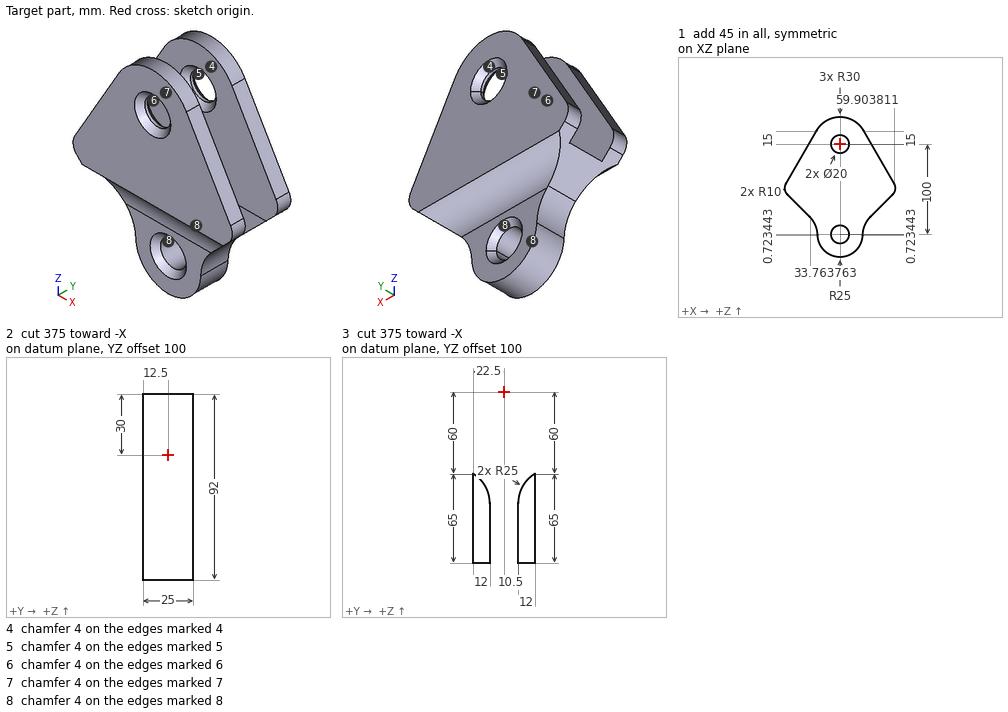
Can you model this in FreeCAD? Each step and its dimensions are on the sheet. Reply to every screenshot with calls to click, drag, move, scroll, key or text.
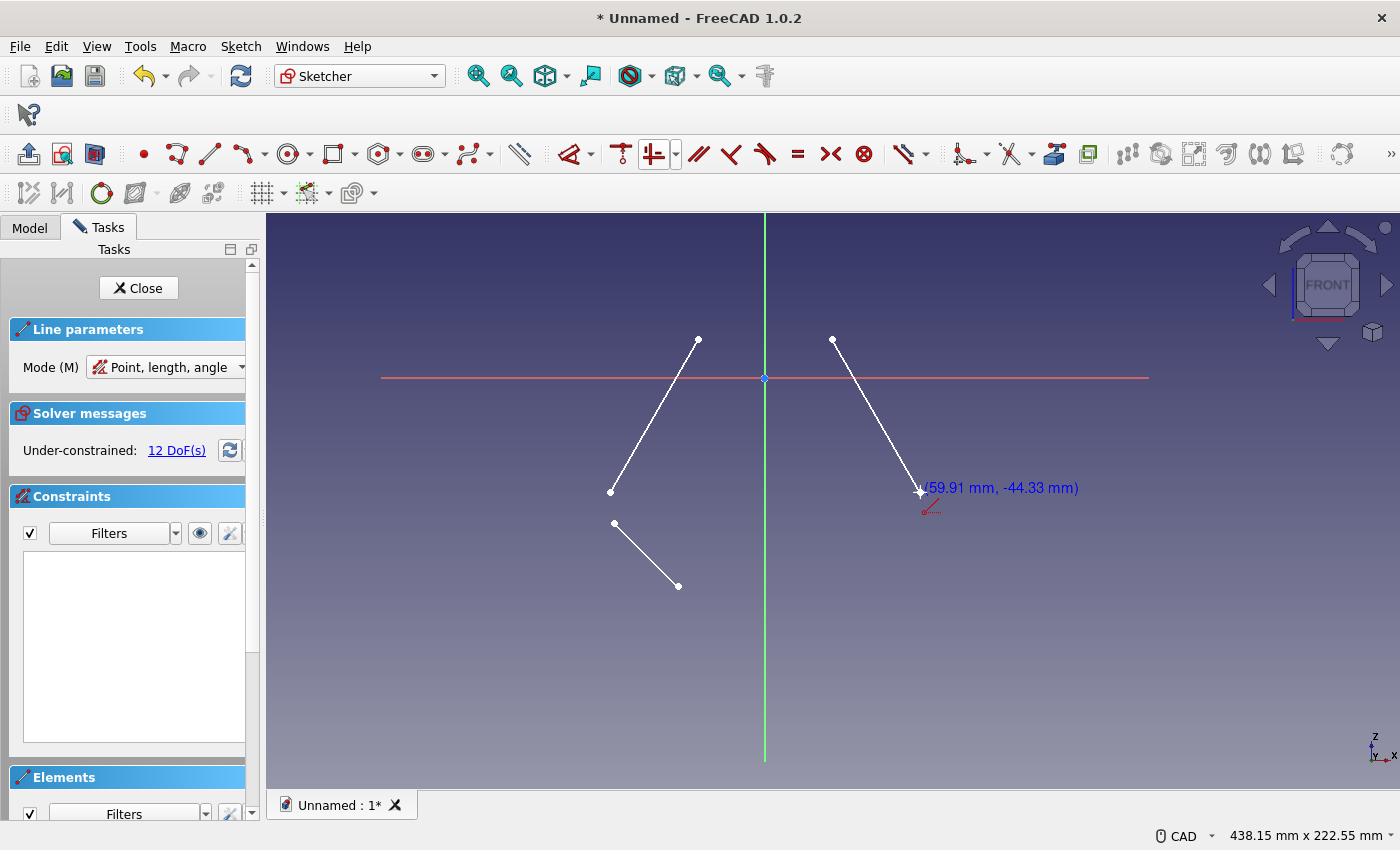
click(916, 523)
click(852, 586)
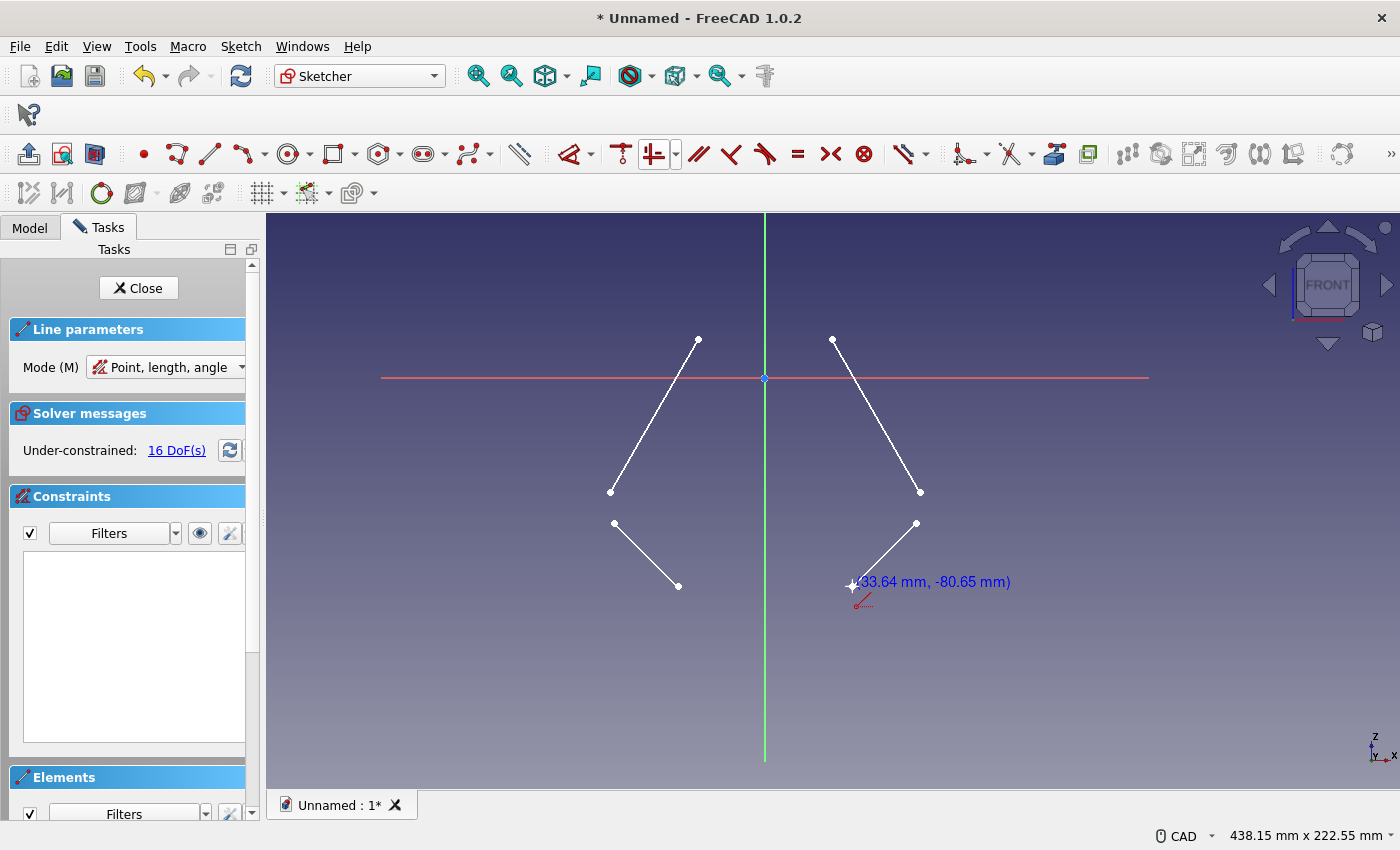
click(242, 154)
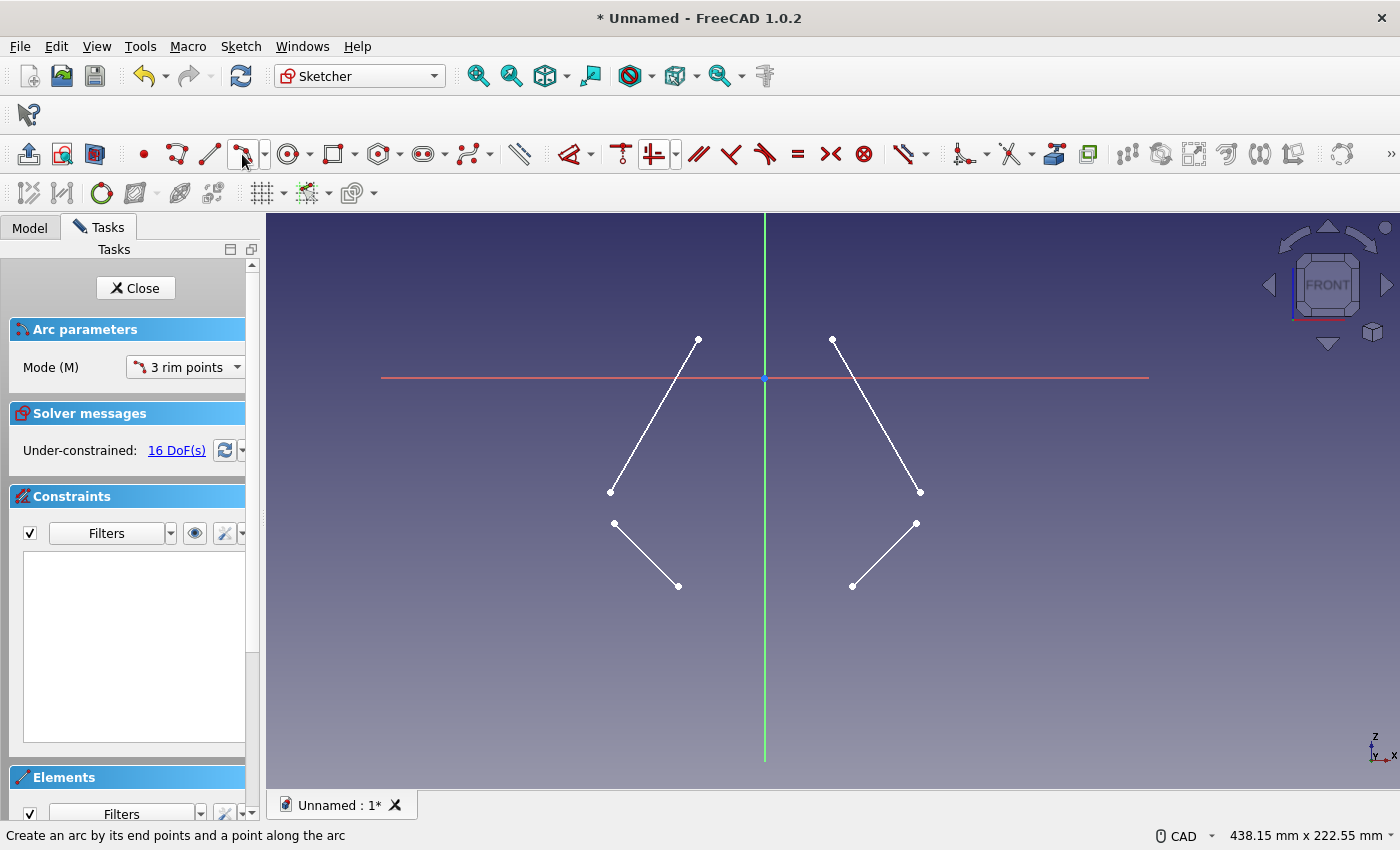
click(614, 524)
click(610, 493)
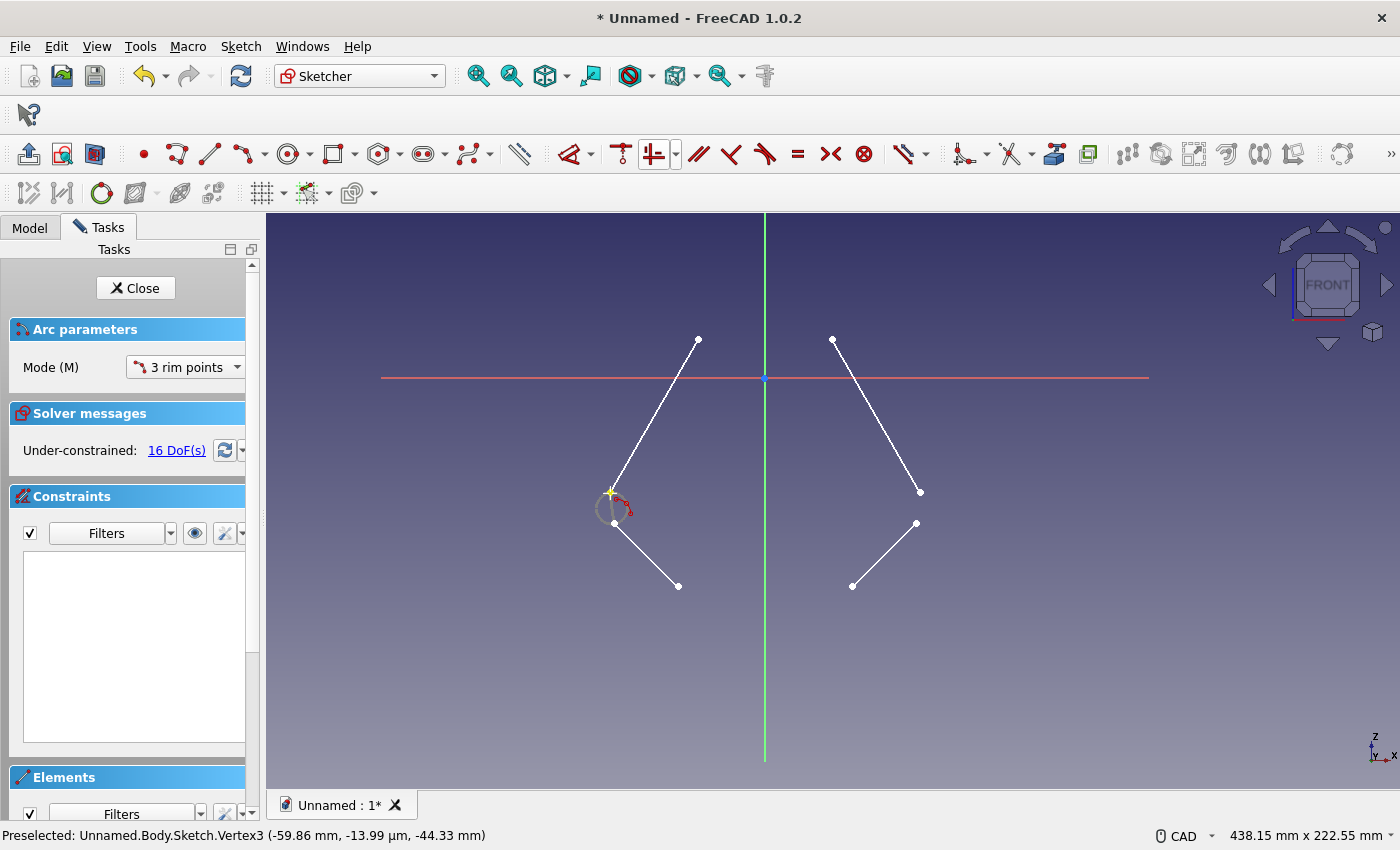
scroll(607, 508, up, 6)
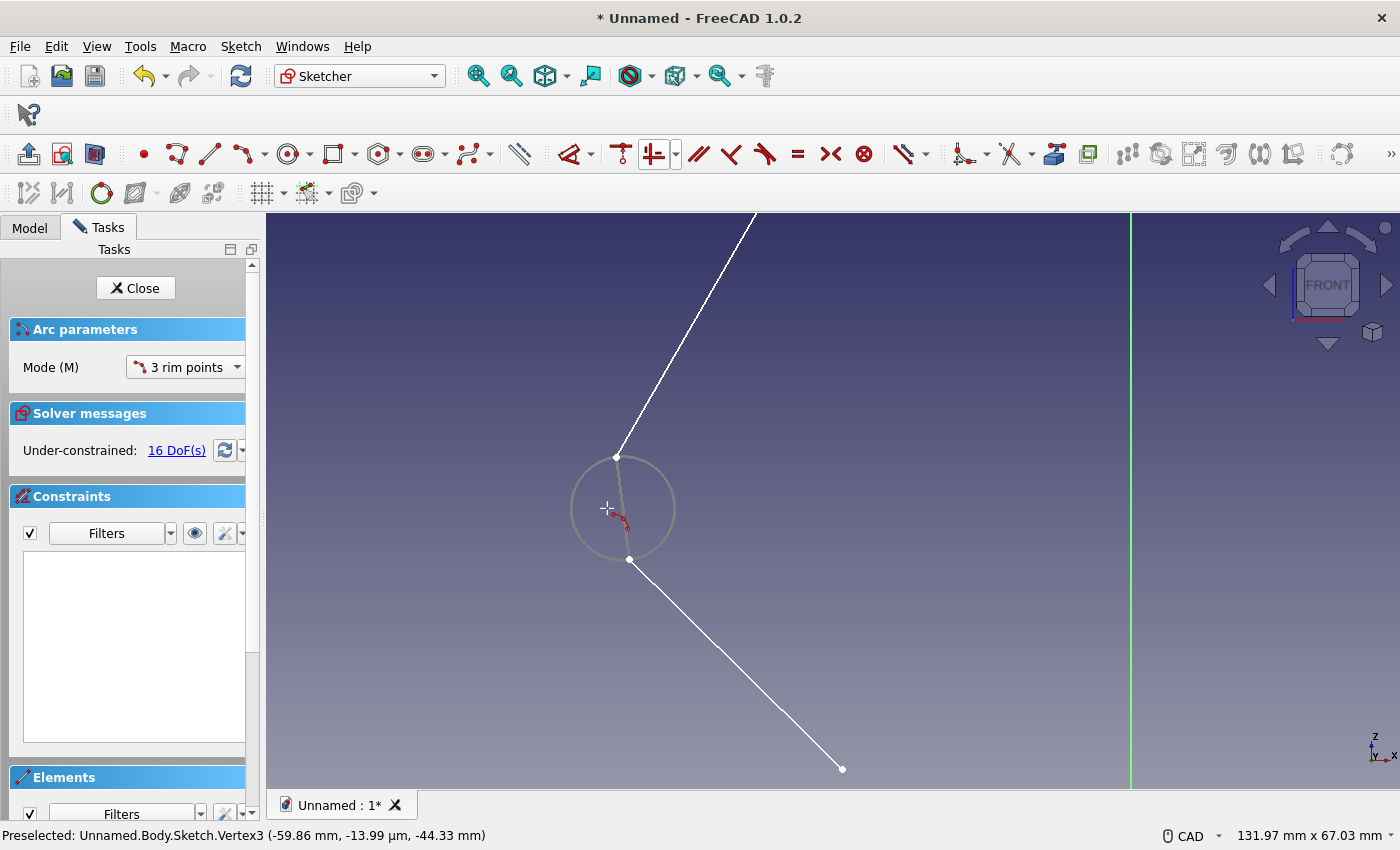
click(605, 506)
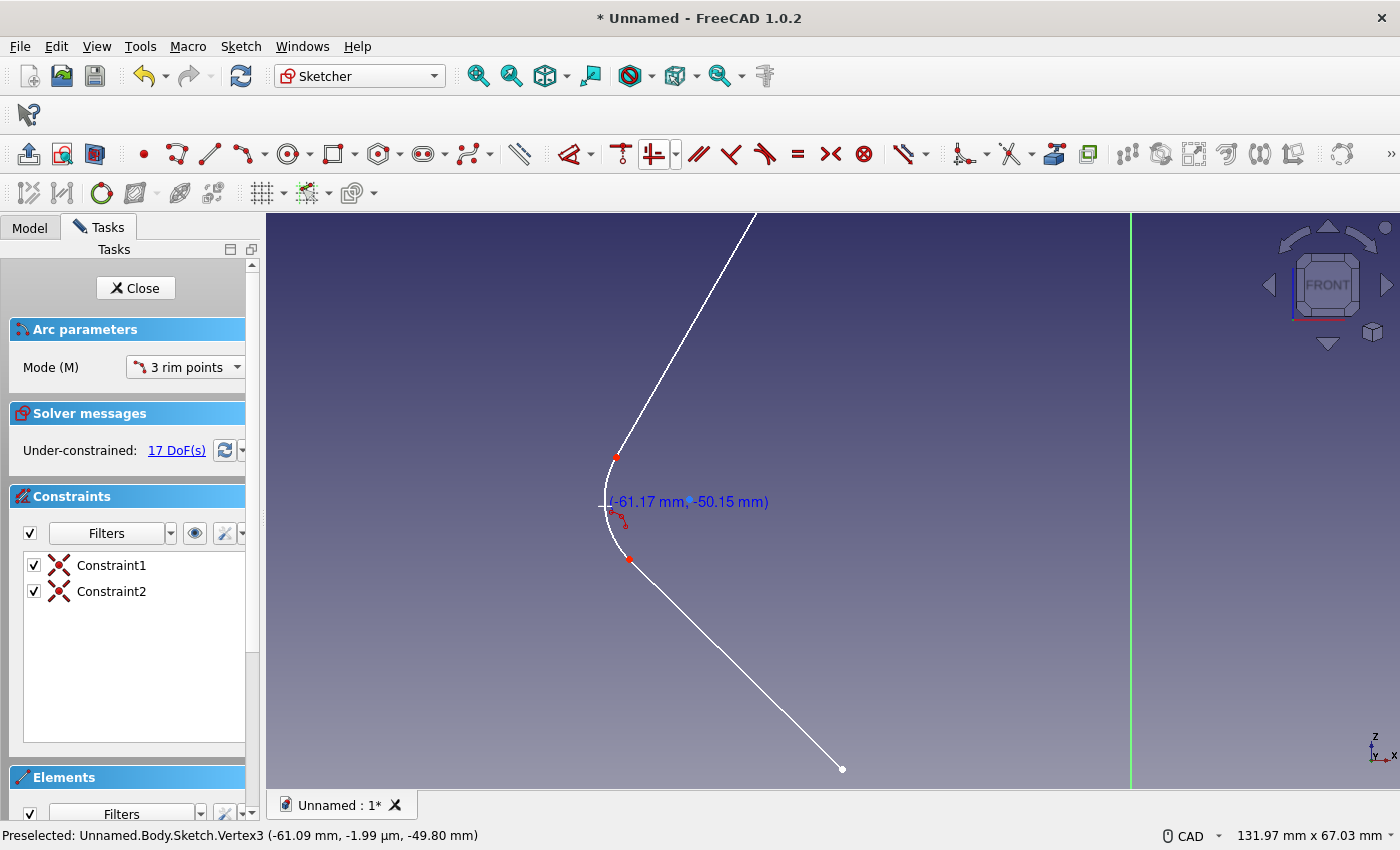
scroll(607, 508, down, 6)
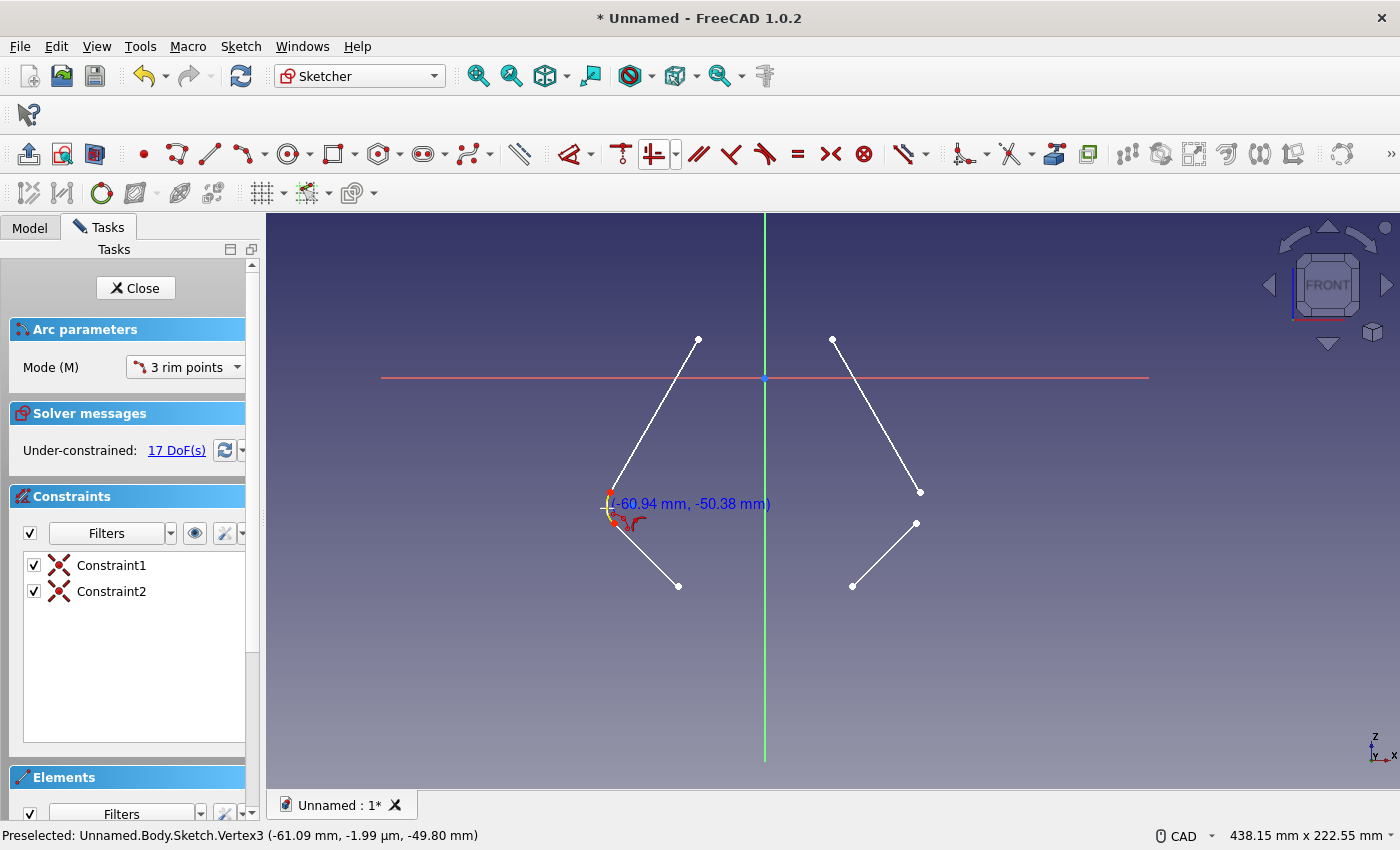
click(698, 340)
click(832, 340)
click(781, 302)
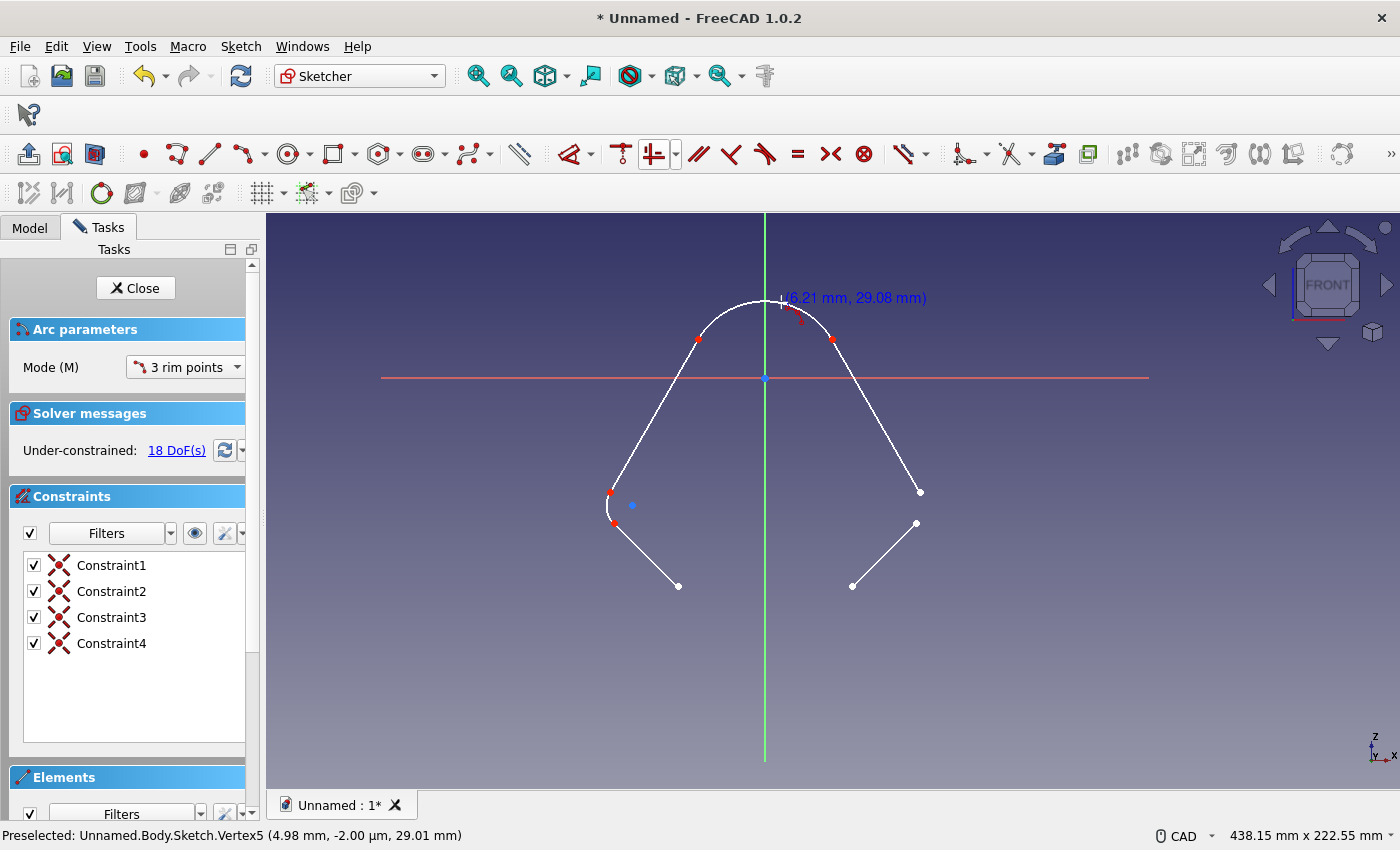
click(920, 493)
click(916, 524)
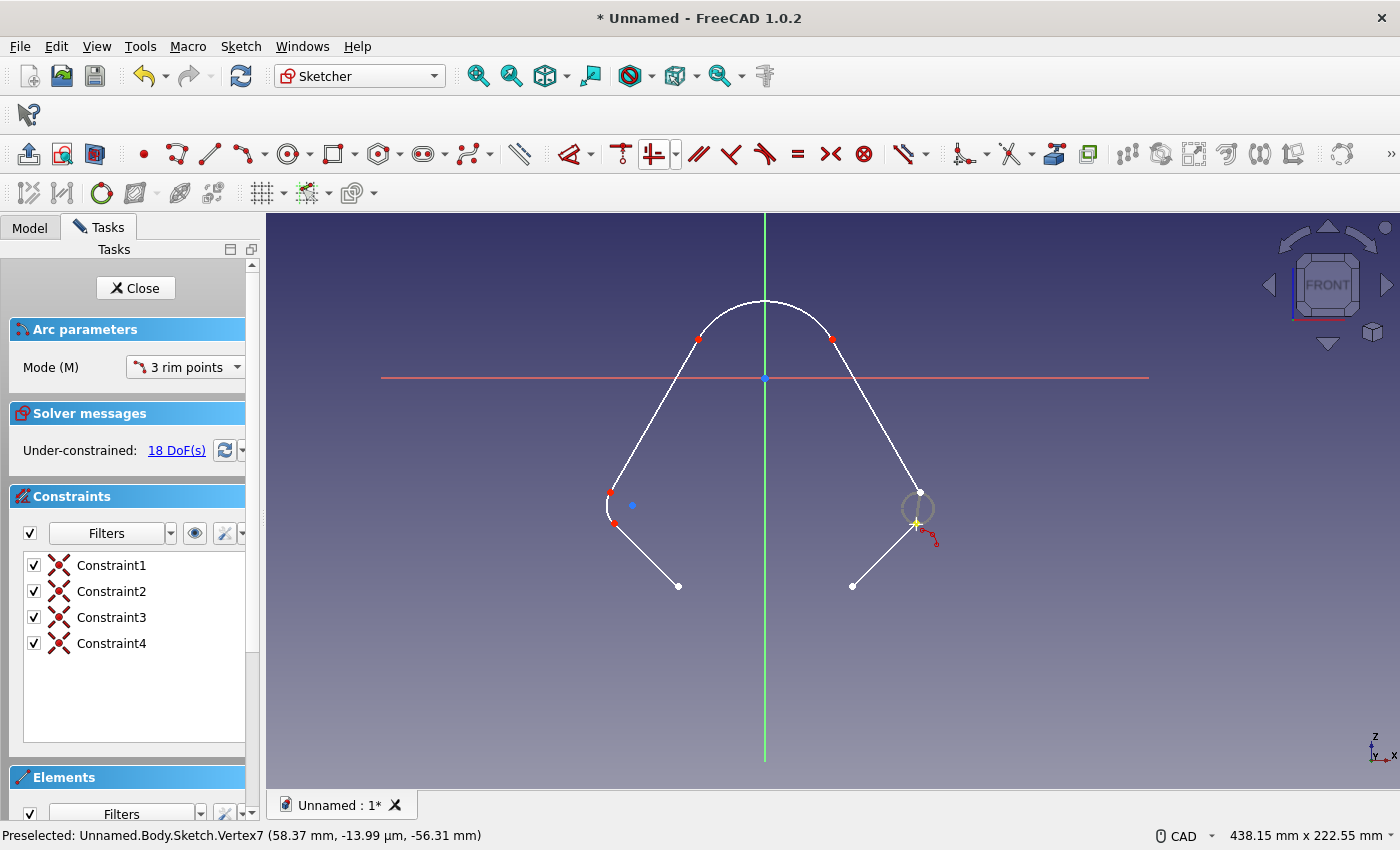
scroll(923, 508, up, 6)